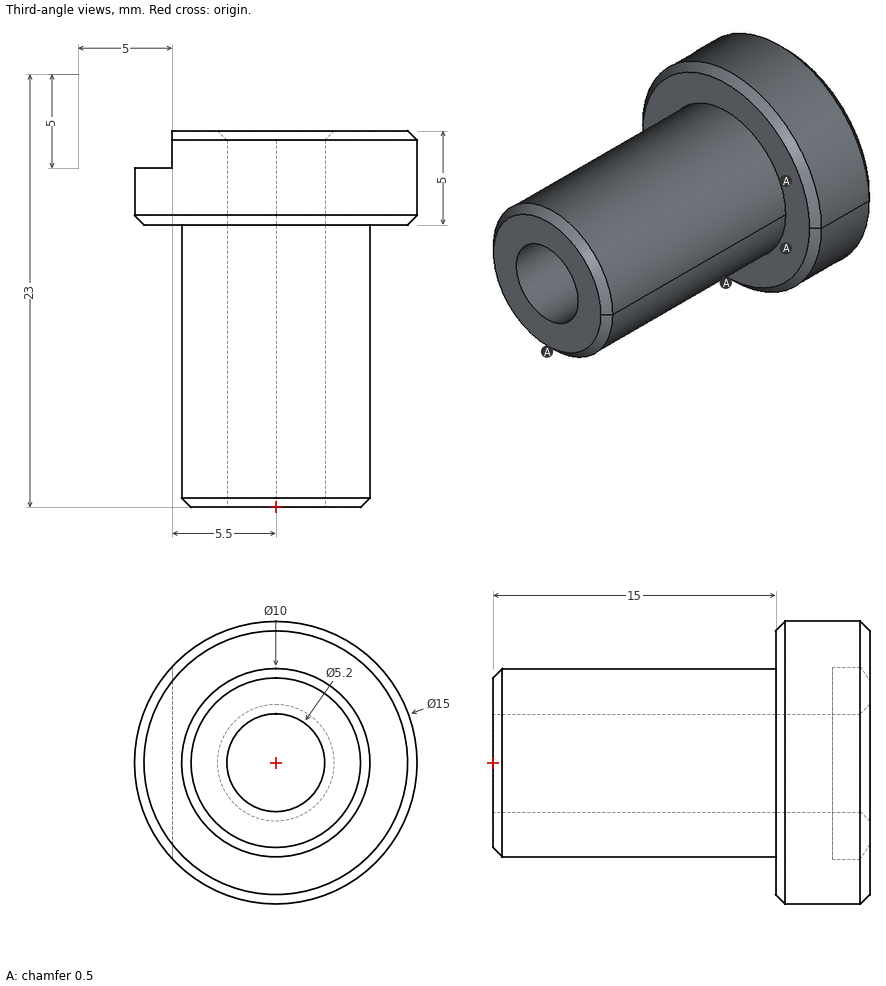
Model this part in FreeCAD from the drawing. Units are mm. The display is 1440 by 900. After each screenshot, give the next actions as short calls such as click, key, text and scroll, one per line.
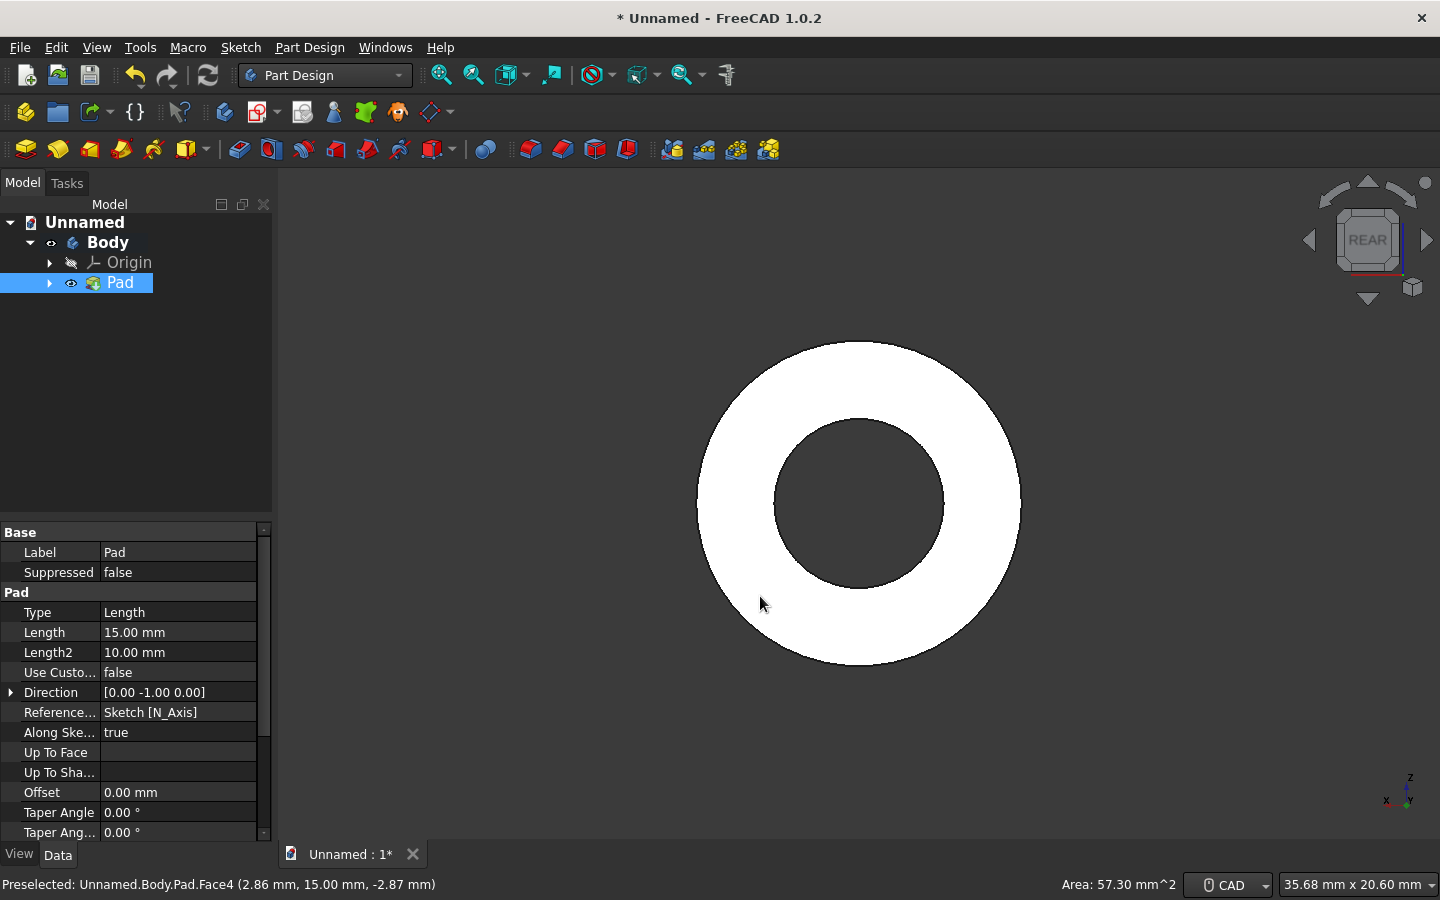
click(258, 112)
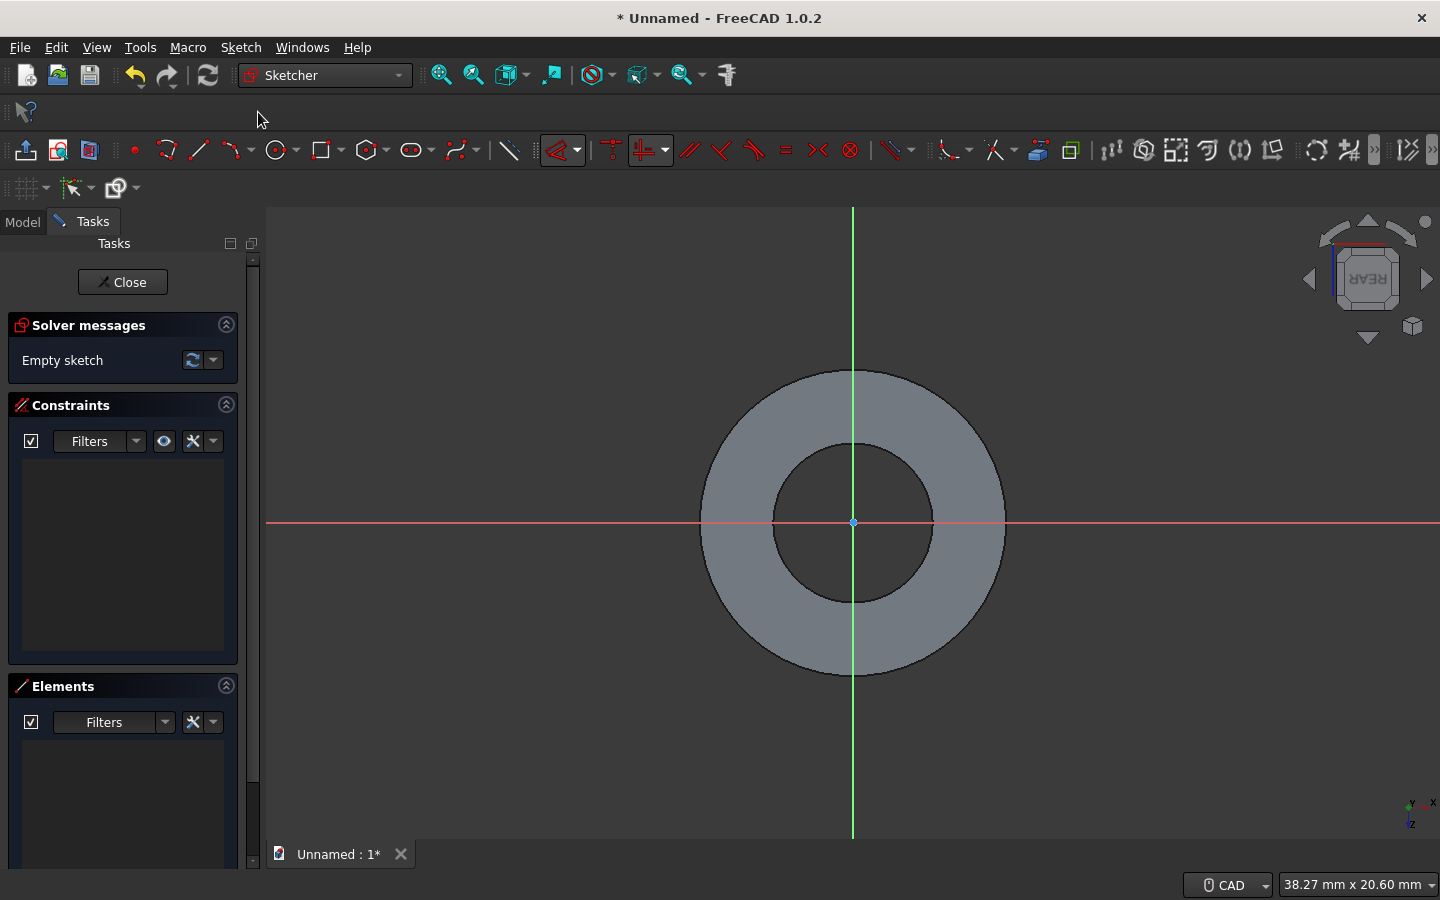
click(276, 150)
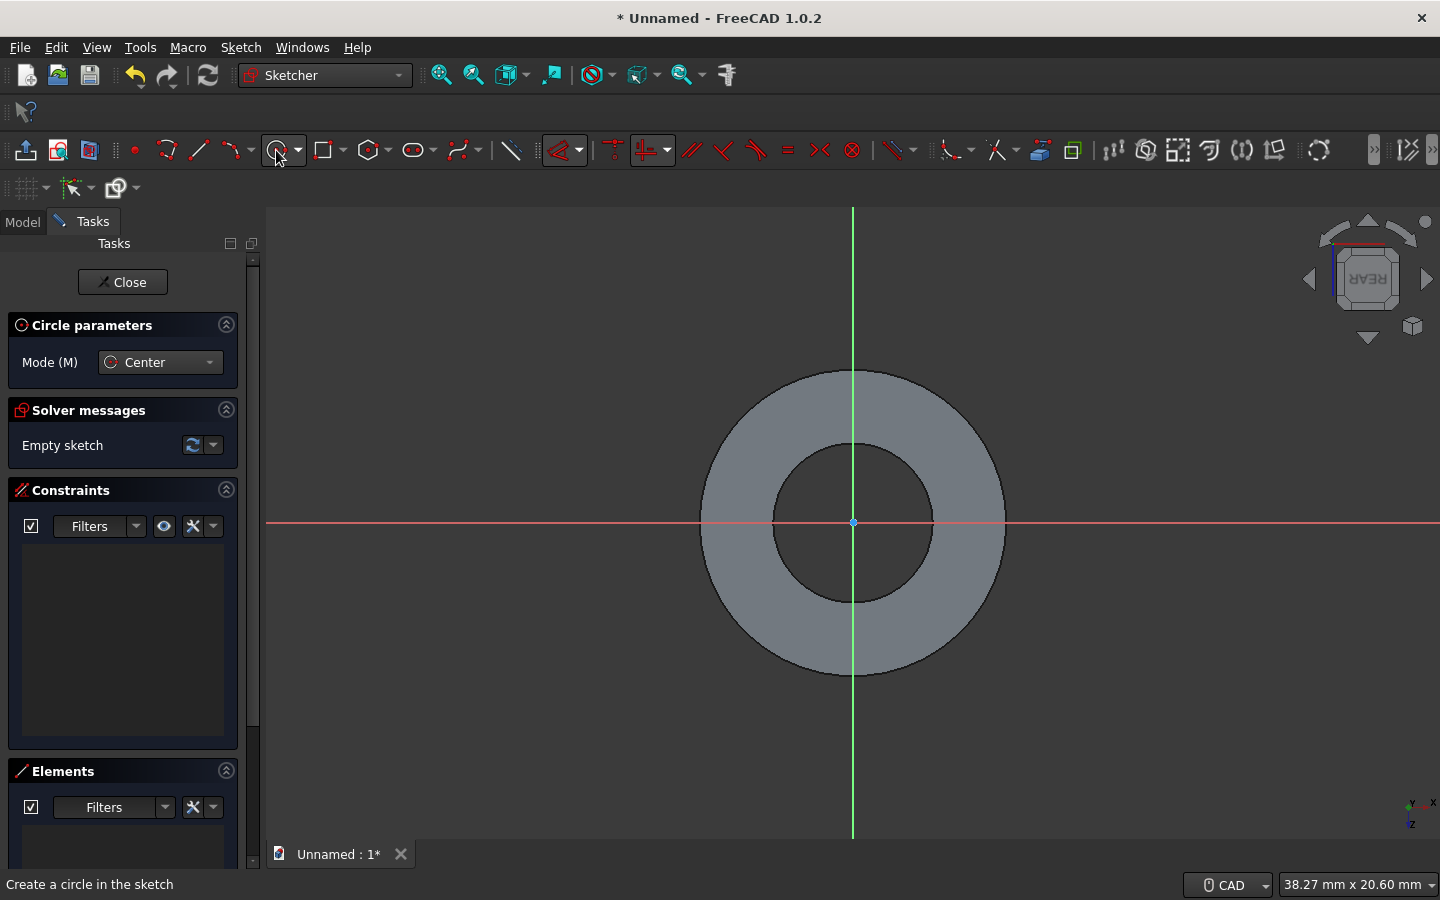
click(853, 523)
click(1016, 360)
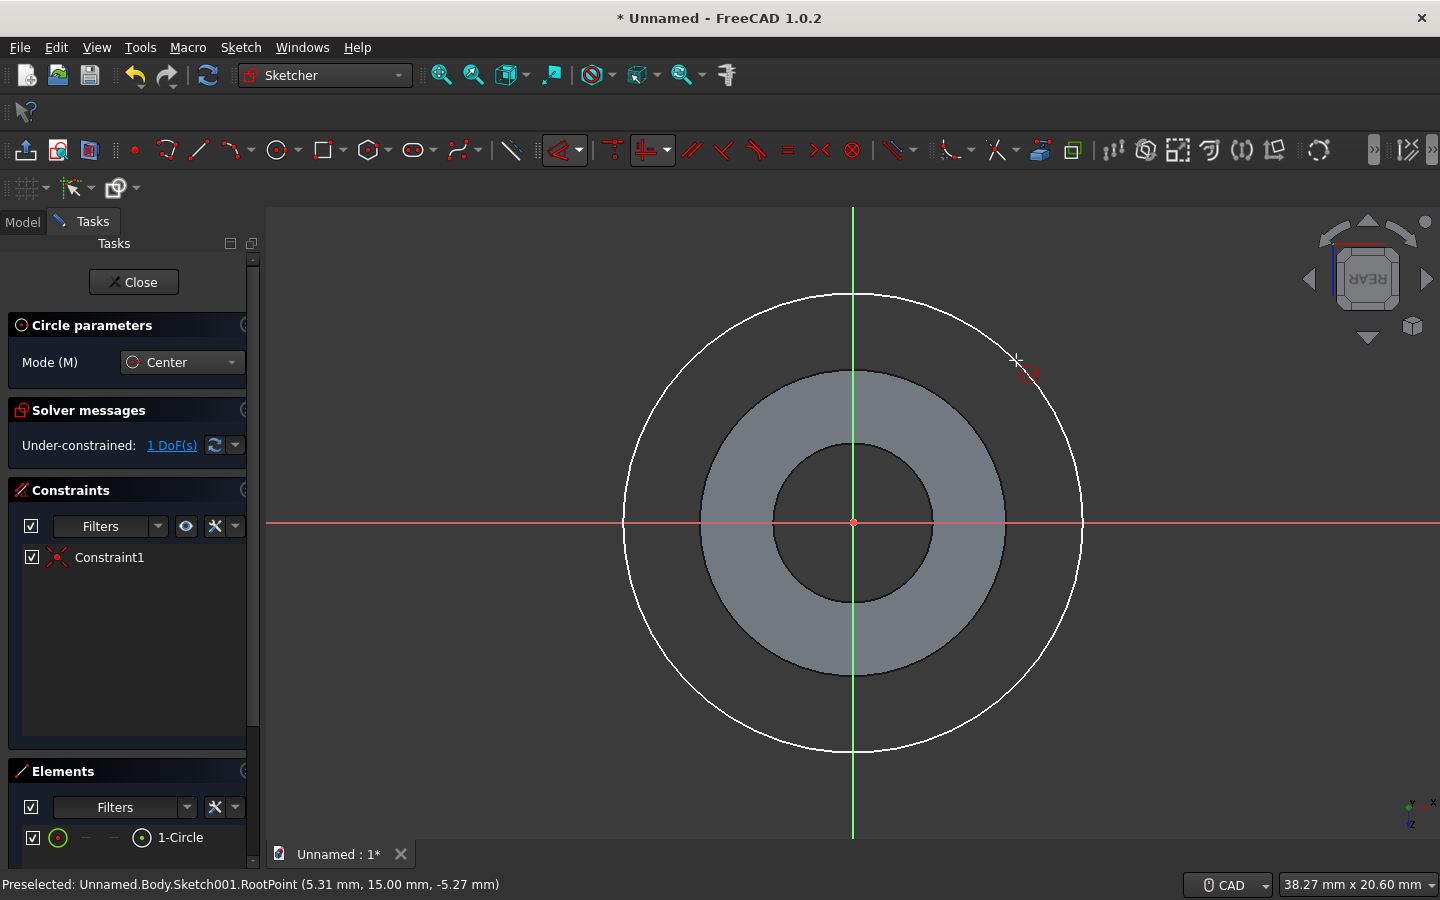
click(853, 523)
click(909, 467)
key(Escape)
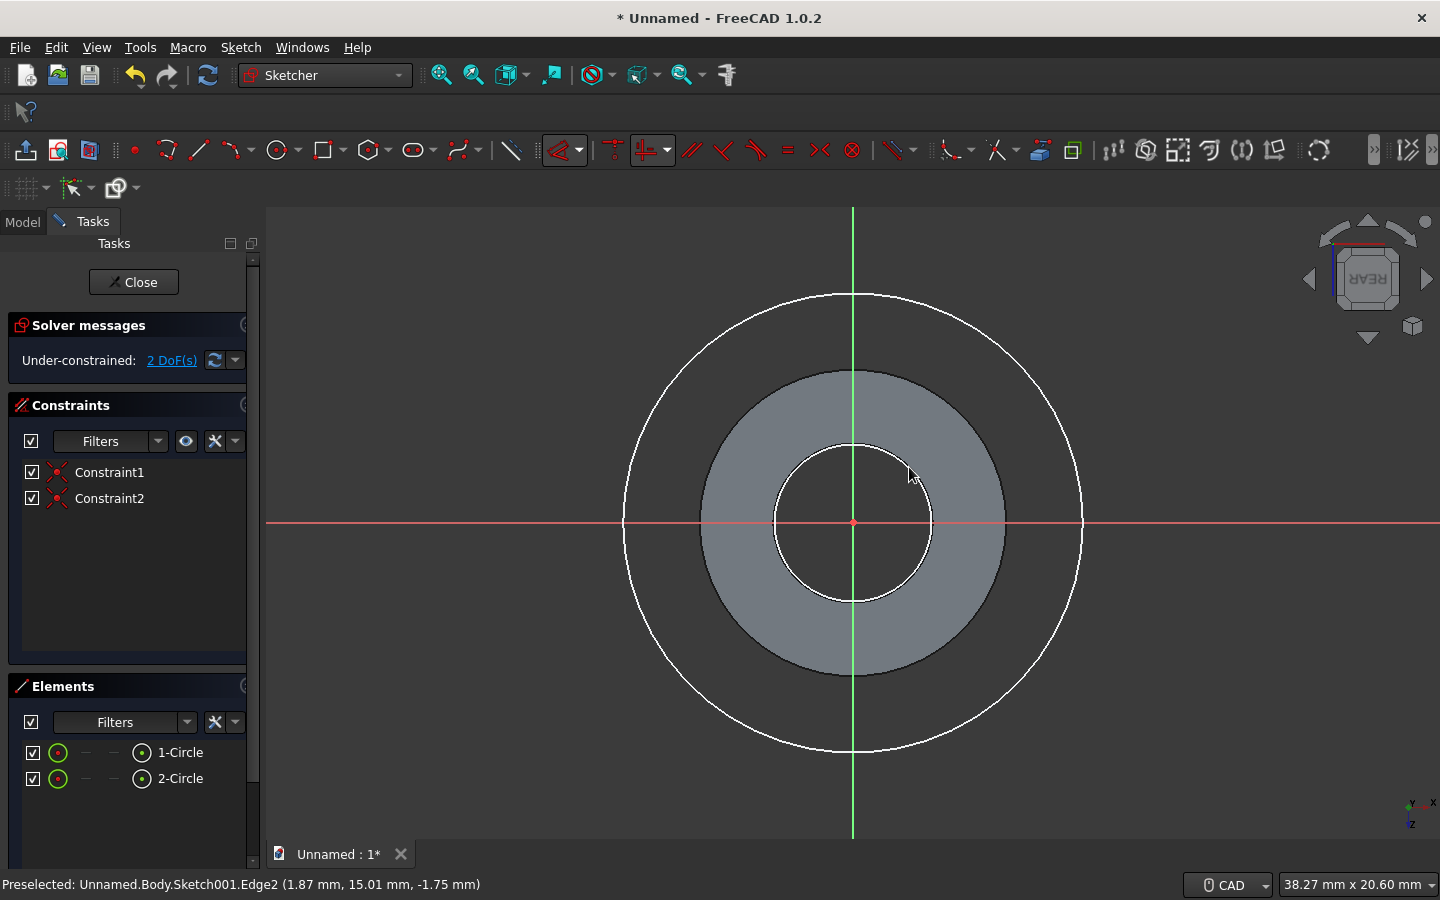
click(1015, 360)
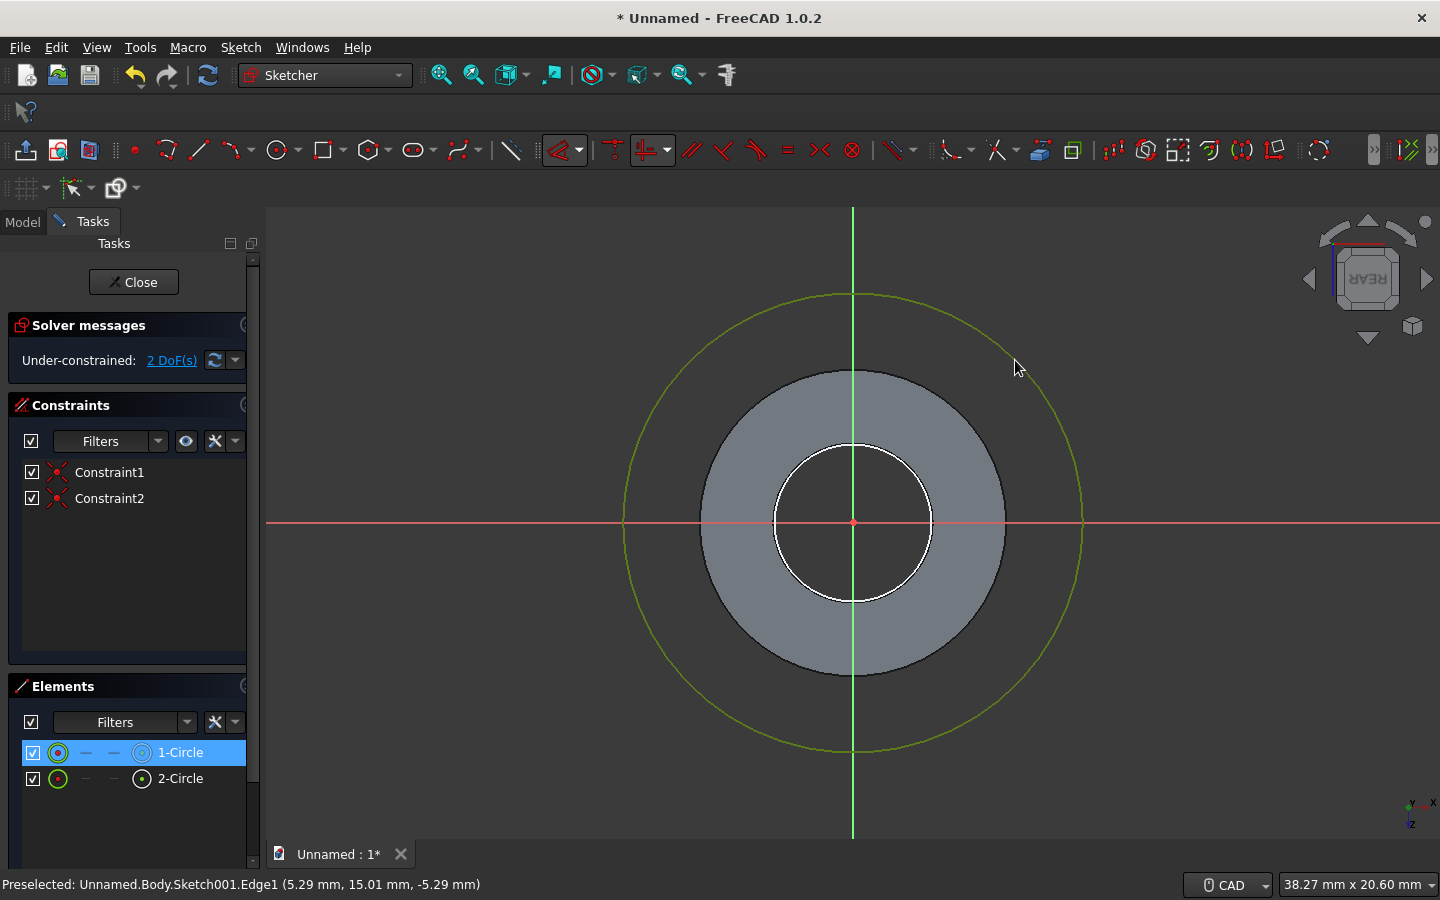
click(582, 150)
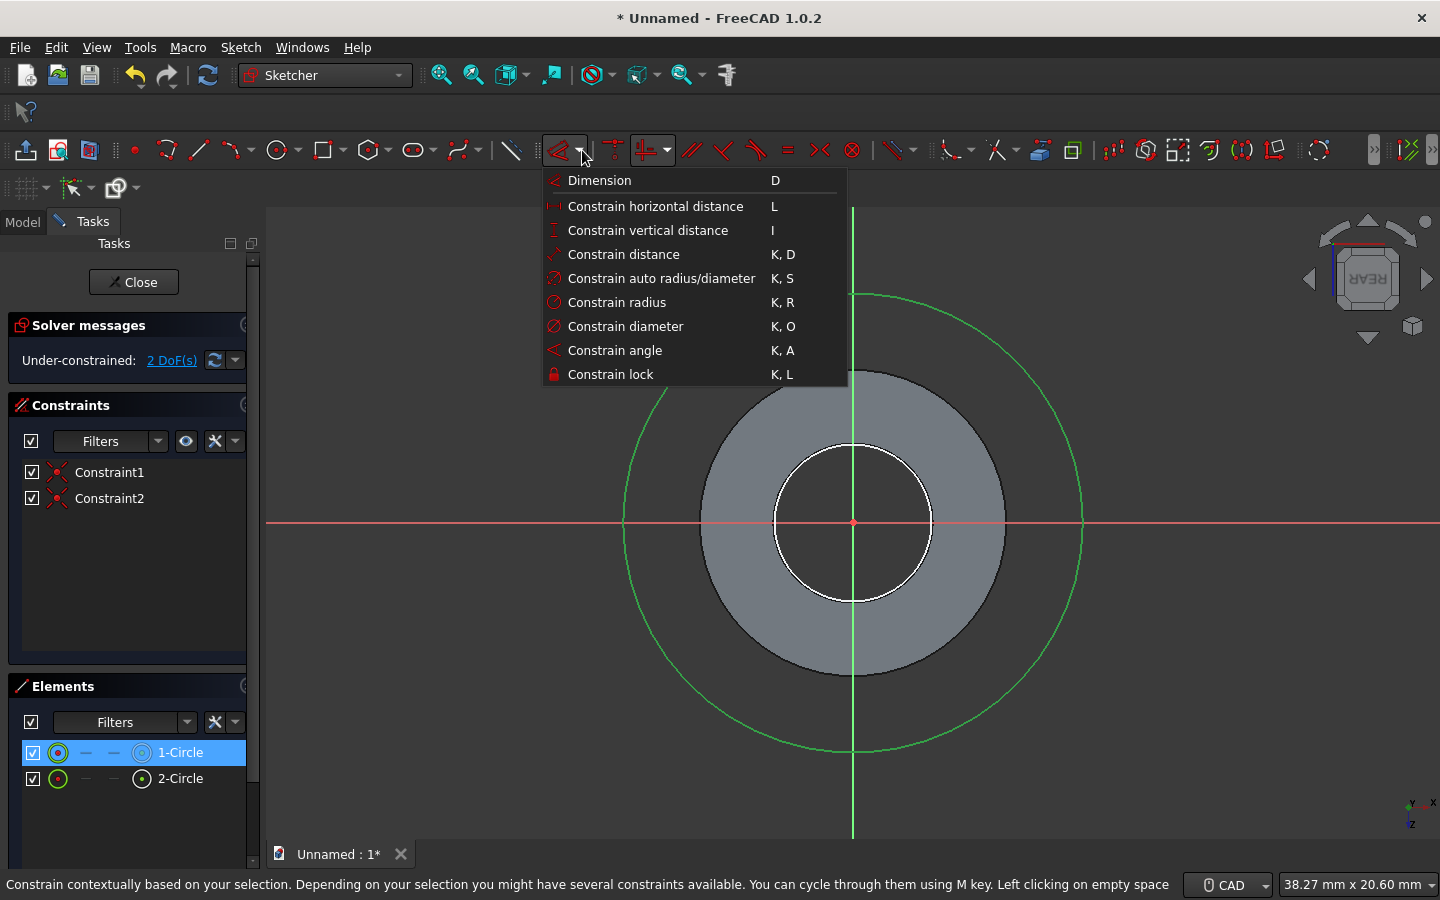
click(695, 326)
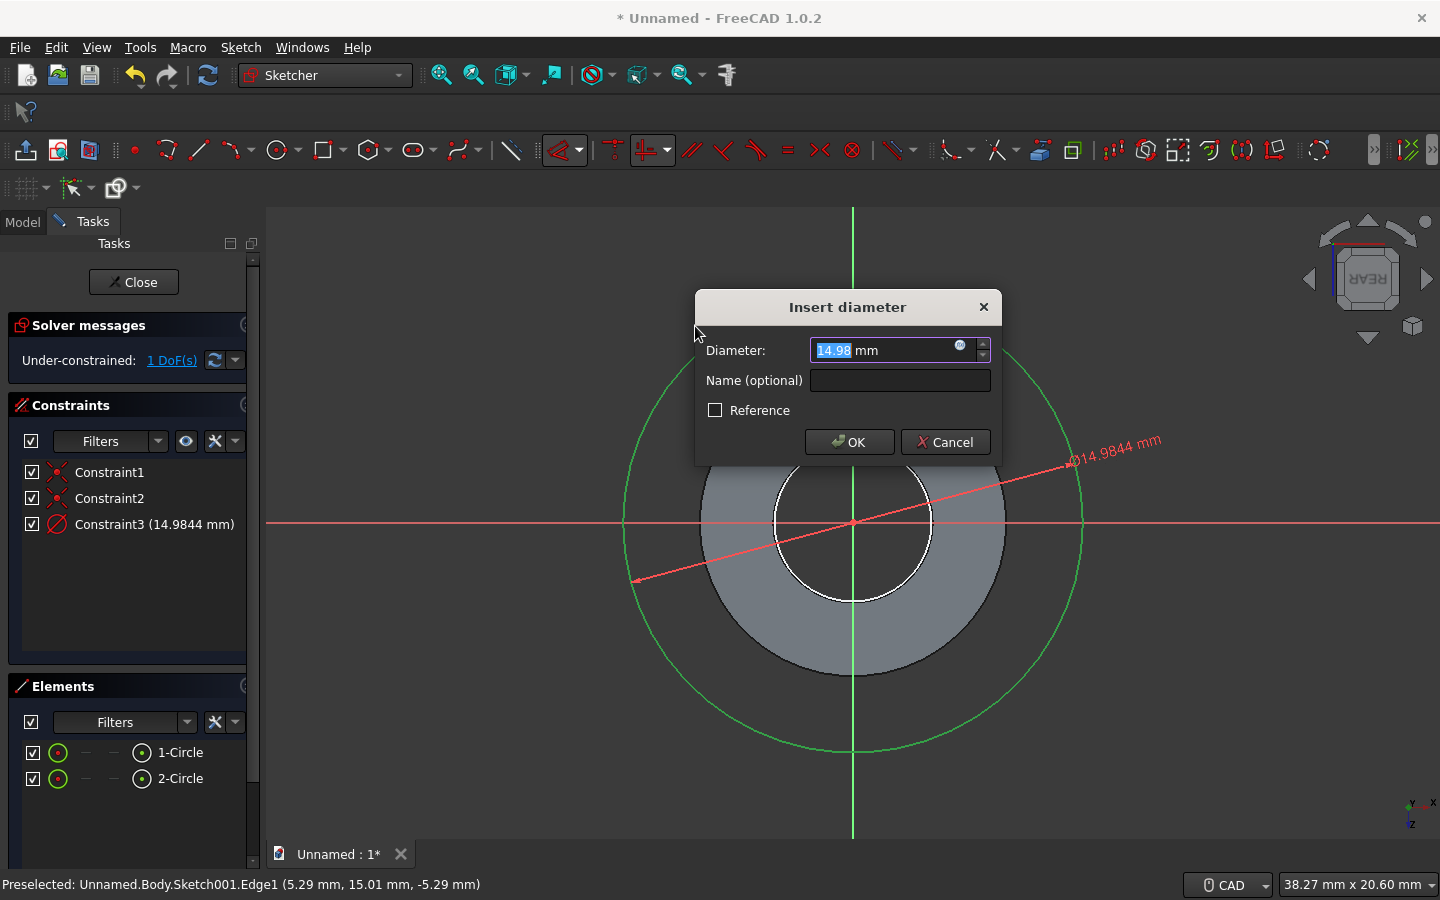
text(15)
key(Return)